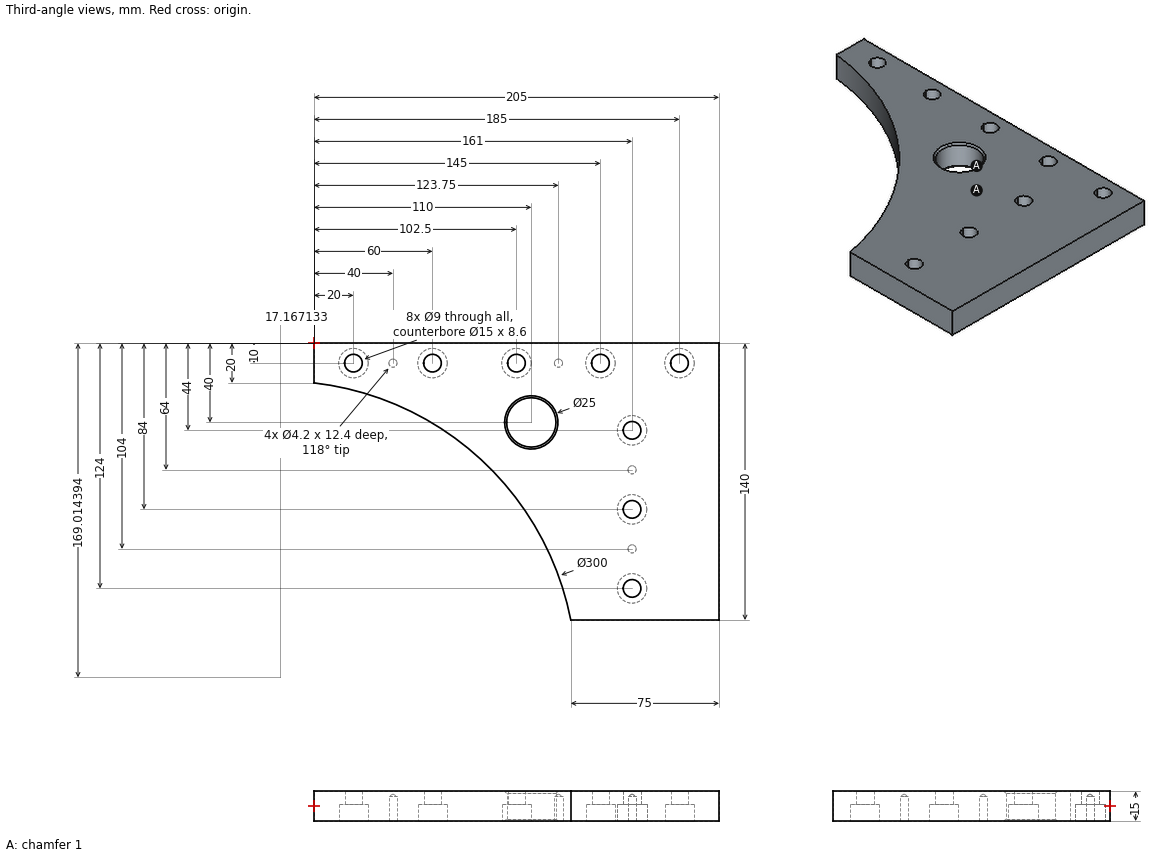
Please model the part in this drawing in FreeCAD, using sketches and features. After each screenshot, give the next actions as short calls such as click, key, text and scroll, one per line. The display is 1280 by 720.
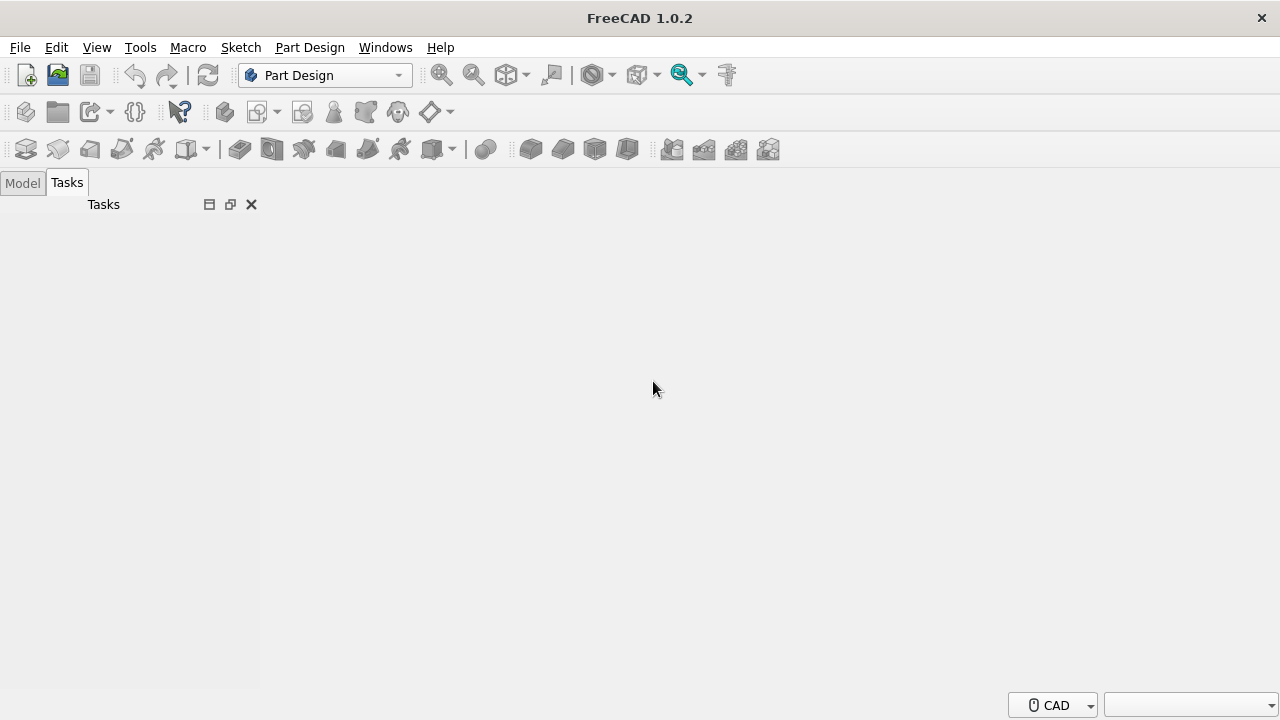
click(26, 76)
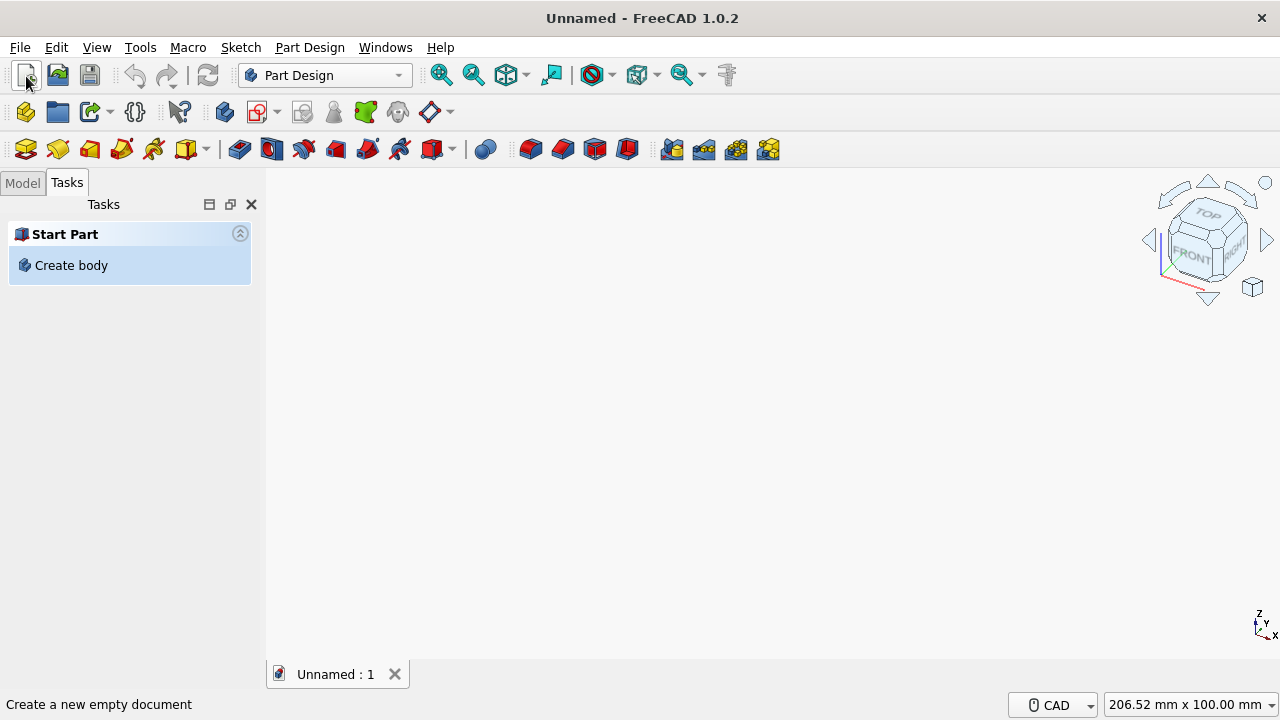
click(258, 112)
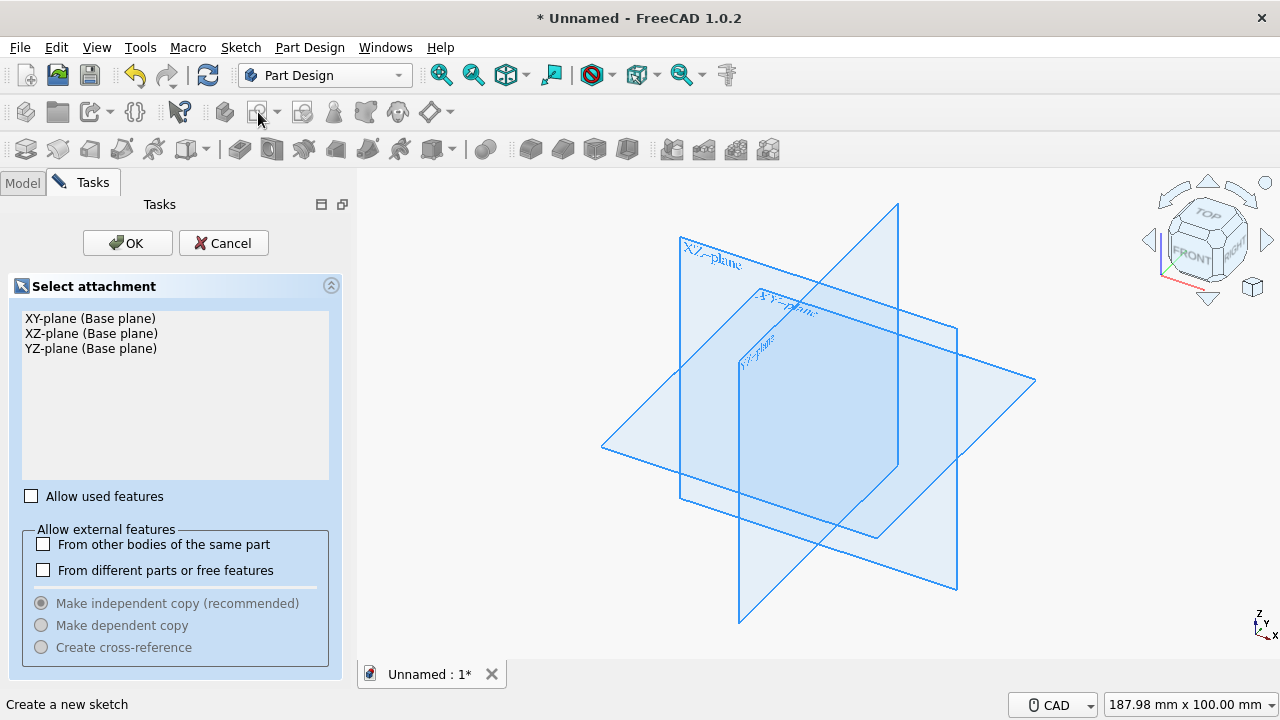
click(82, 318)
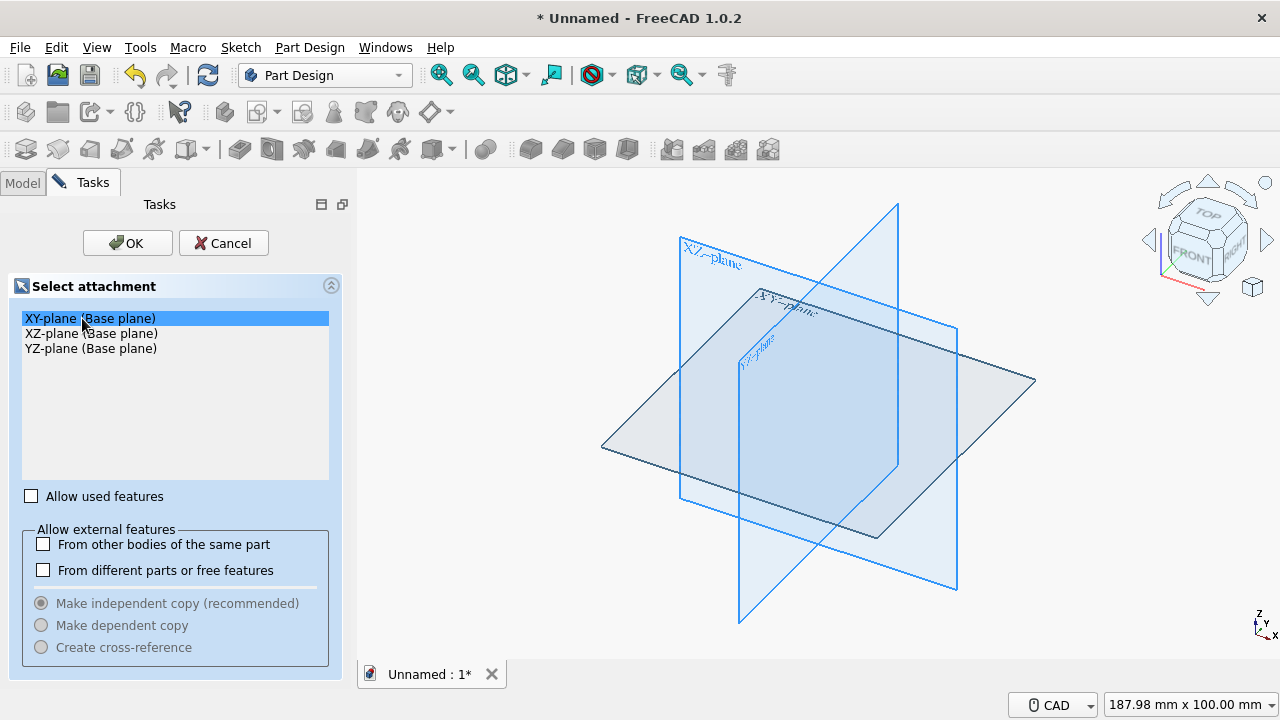
click(128, 243)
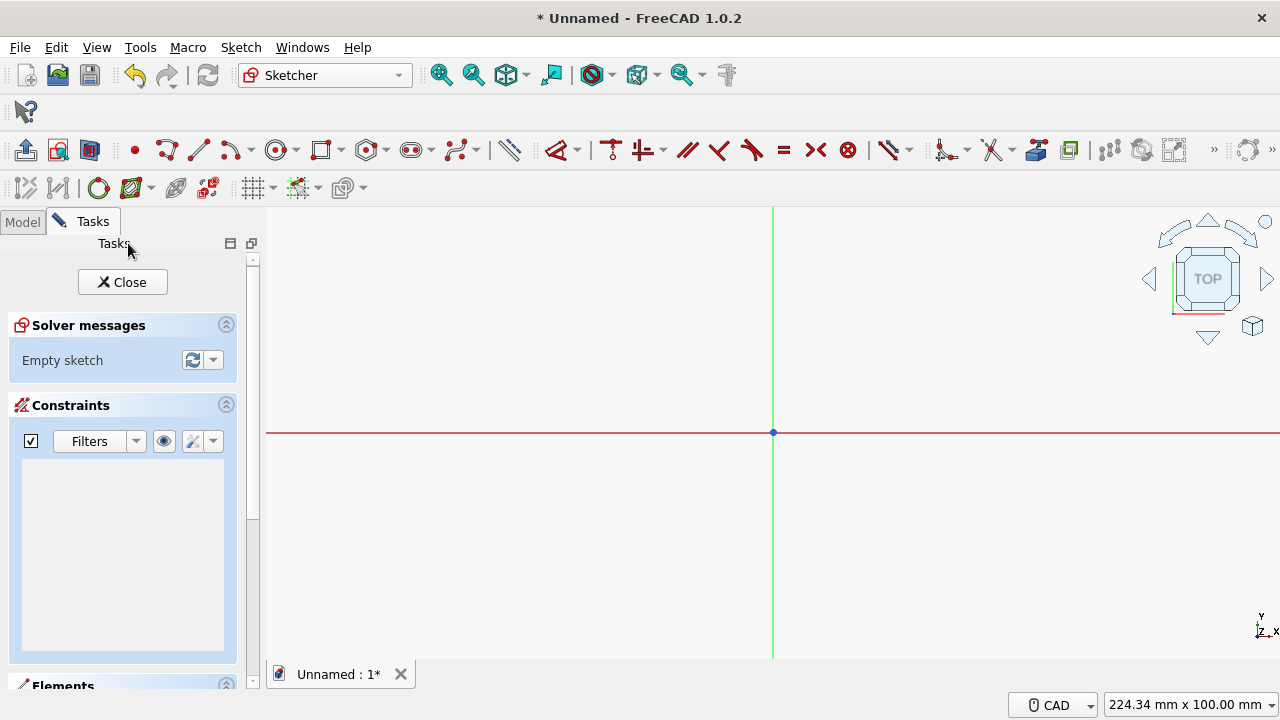
scroll(395, 249, down, 5)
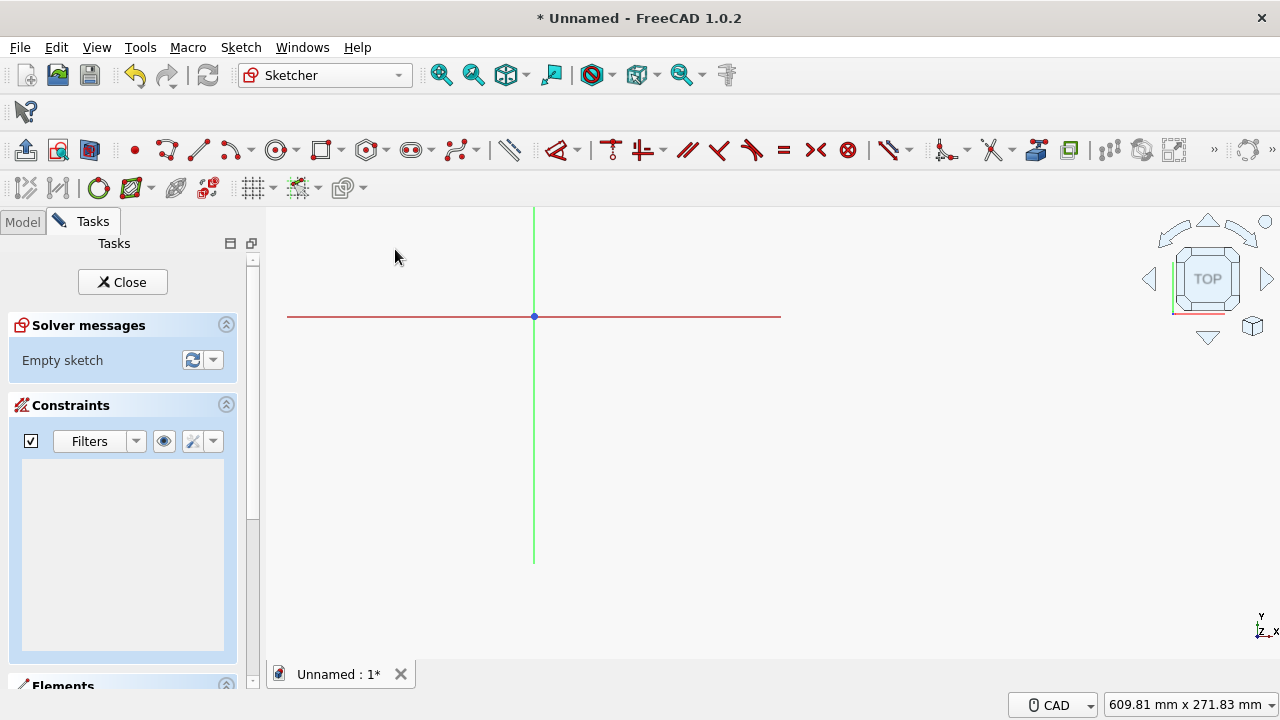
click(168, 150)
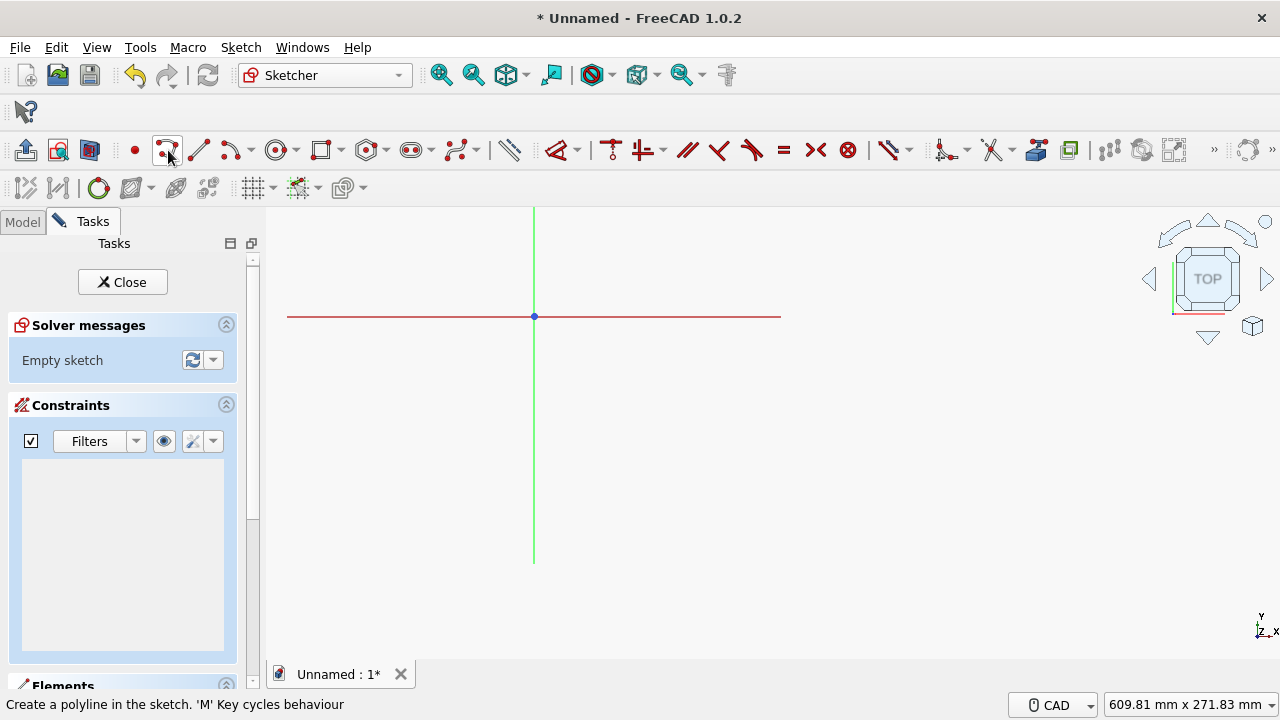
click(534, 317)
click(543, 350)
click(750, 550)
click(875, 550)
click(875, 326)
click(534, 317)
key(Escape)
key(Escape)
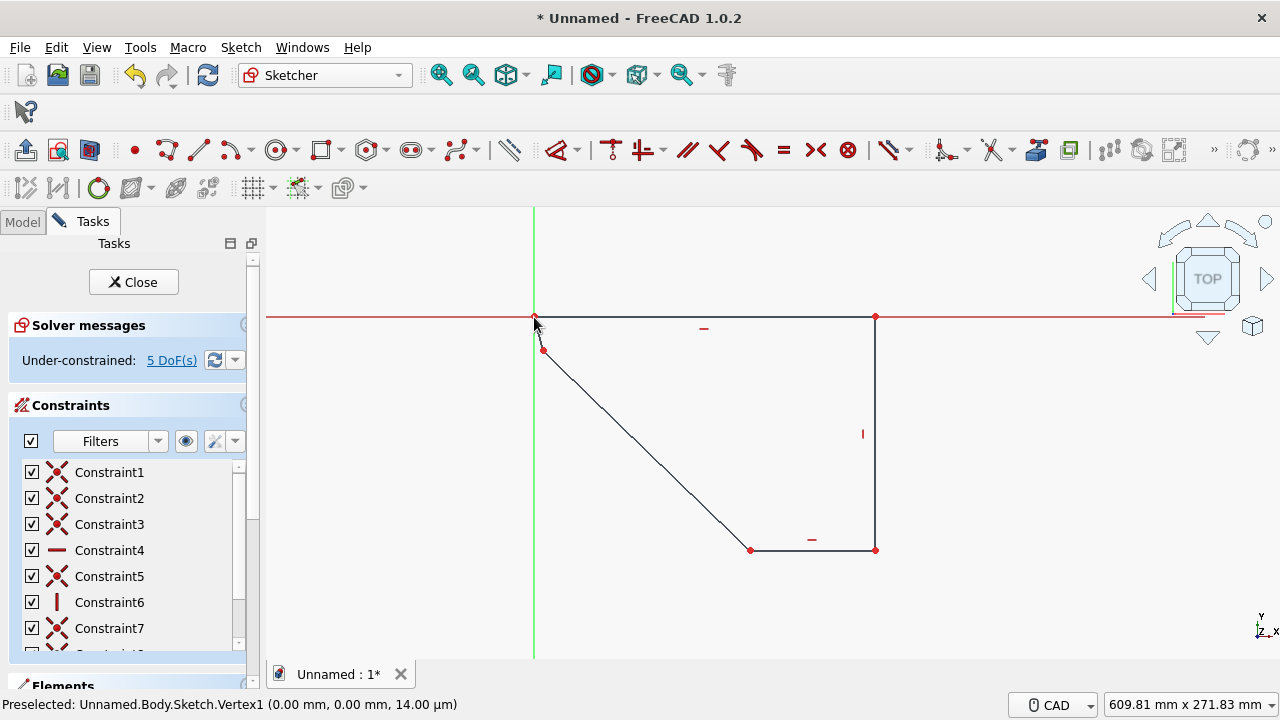
scroll(537, 327, up, 2)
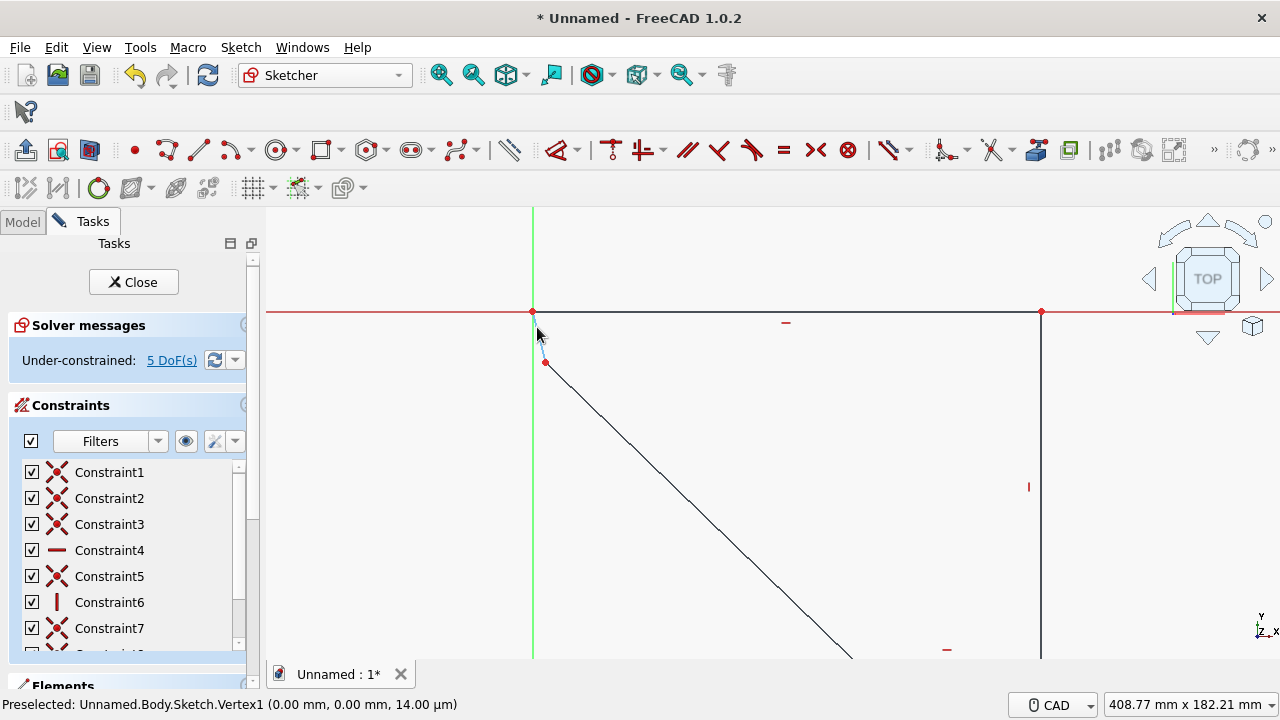
click(537, 327)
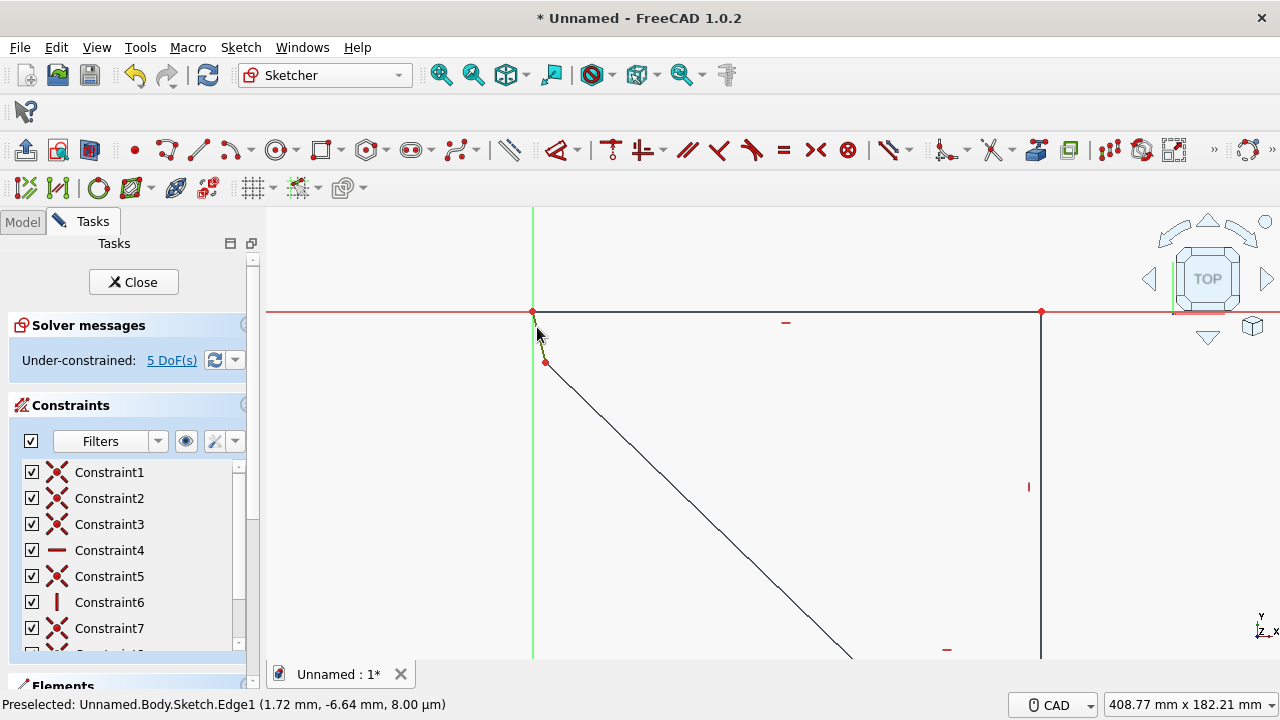
click(666, 150)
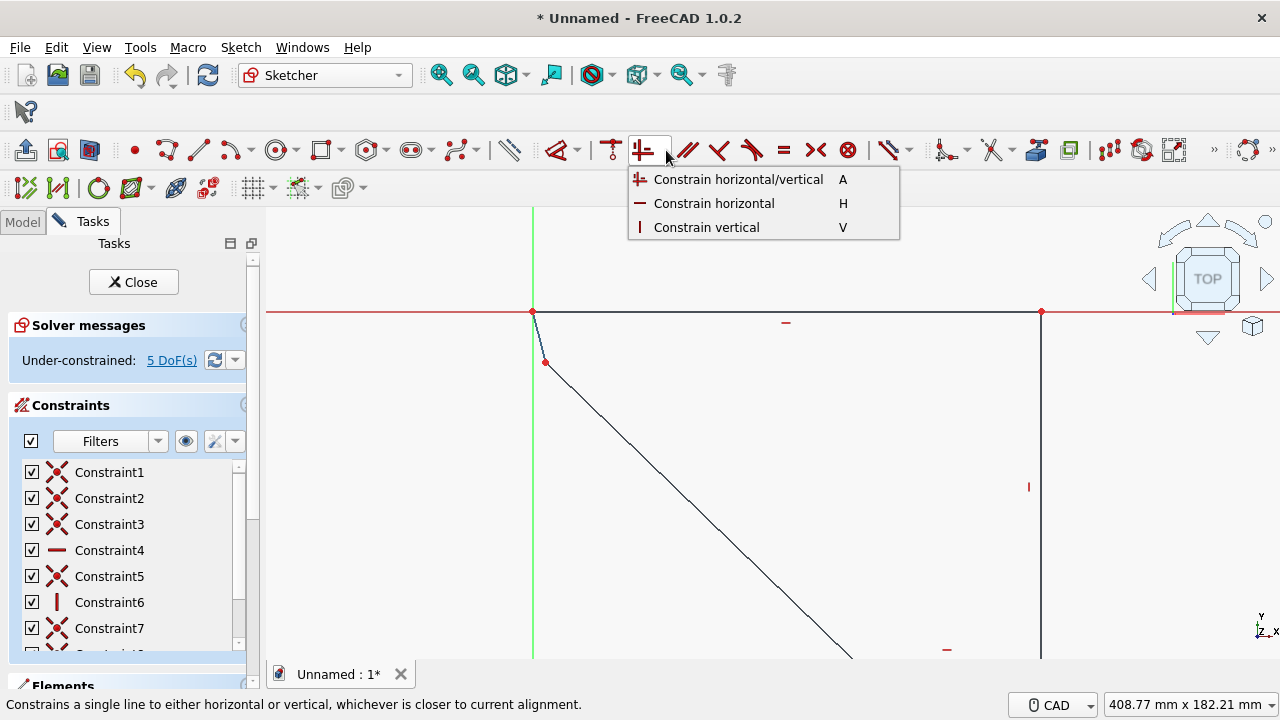
click(764, 227)